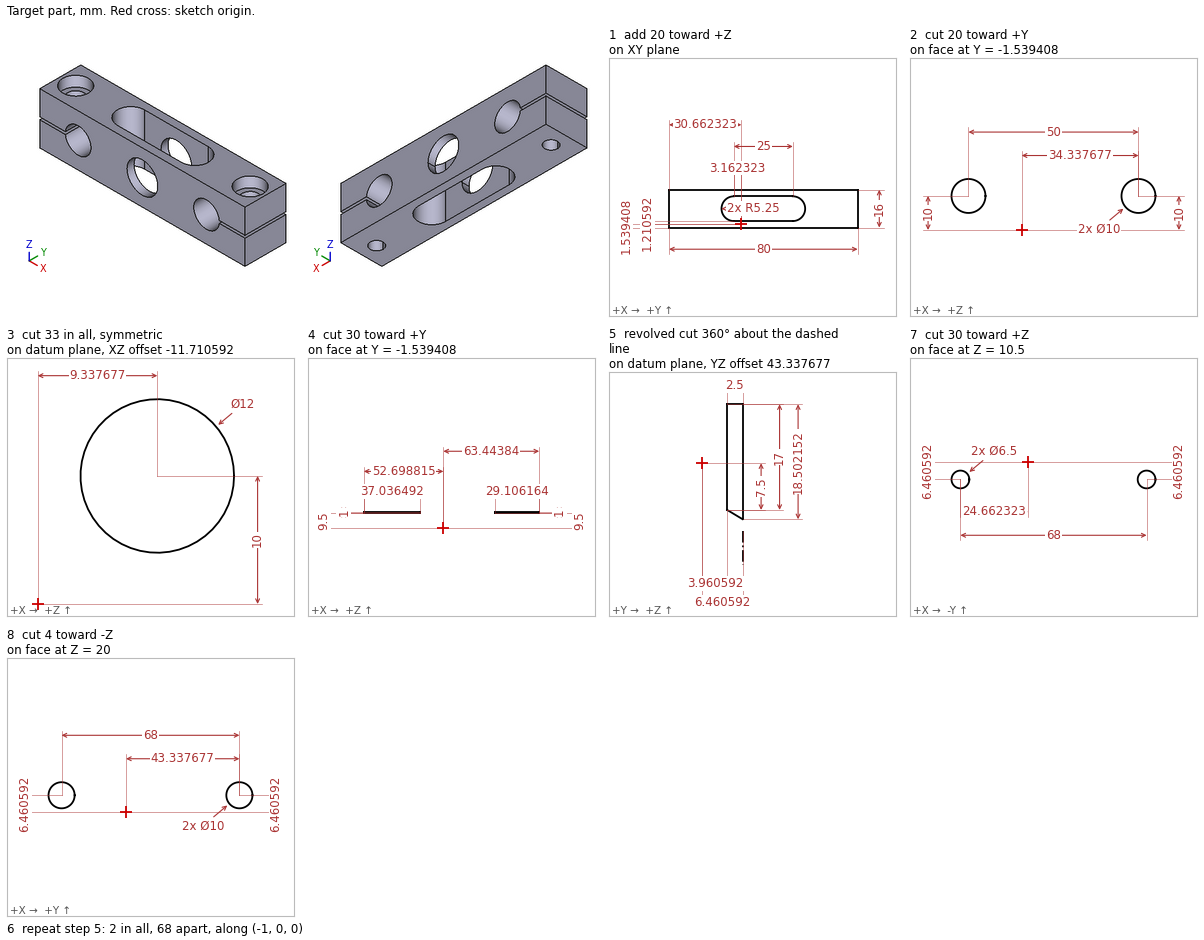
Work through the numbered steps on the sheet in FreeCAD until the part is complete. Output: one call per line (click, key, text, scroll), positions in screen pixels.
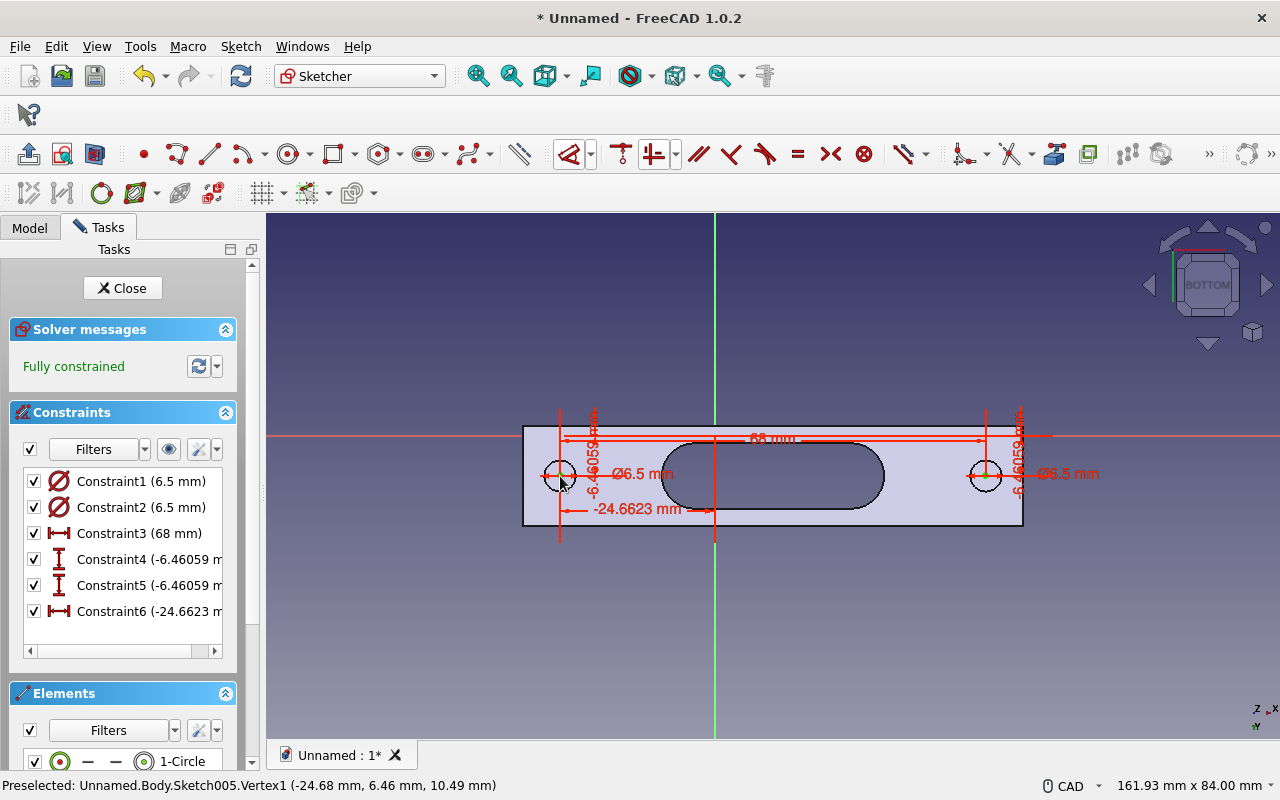
click(123, 288)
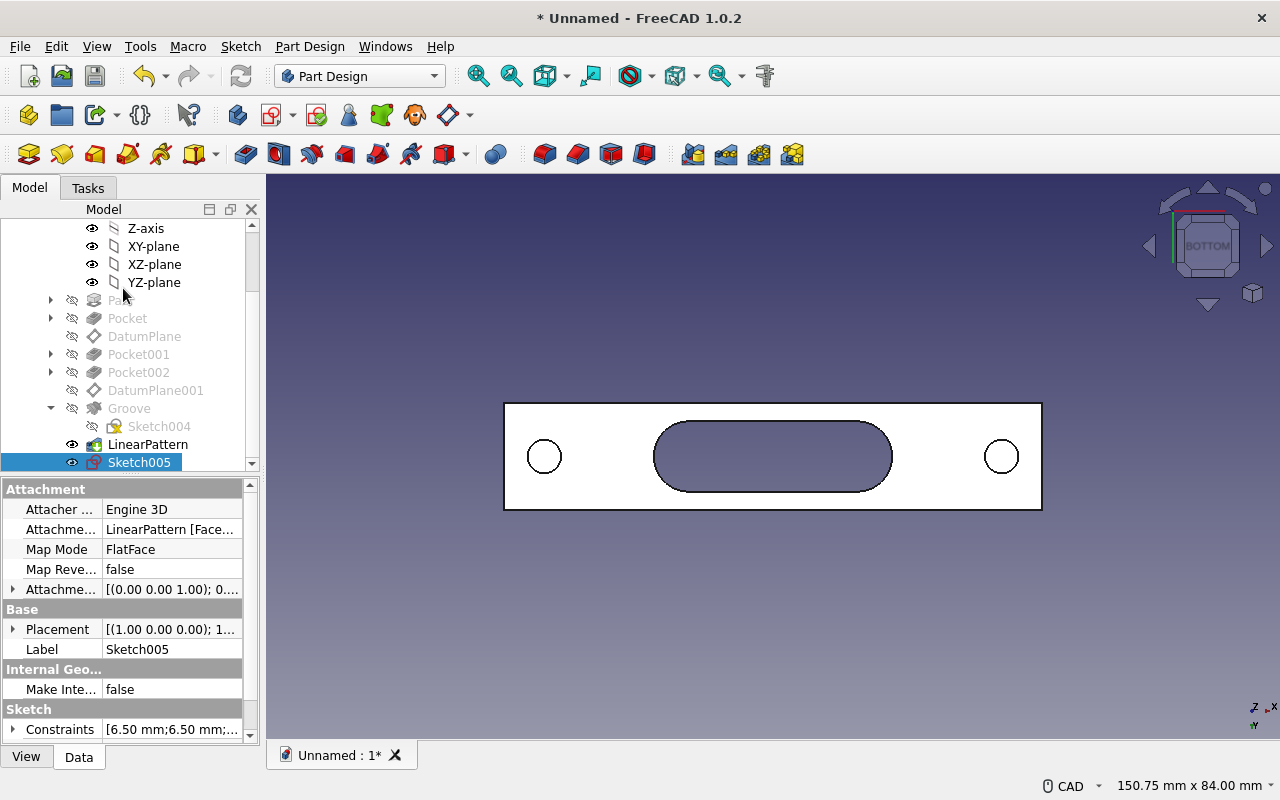
click(246, 154)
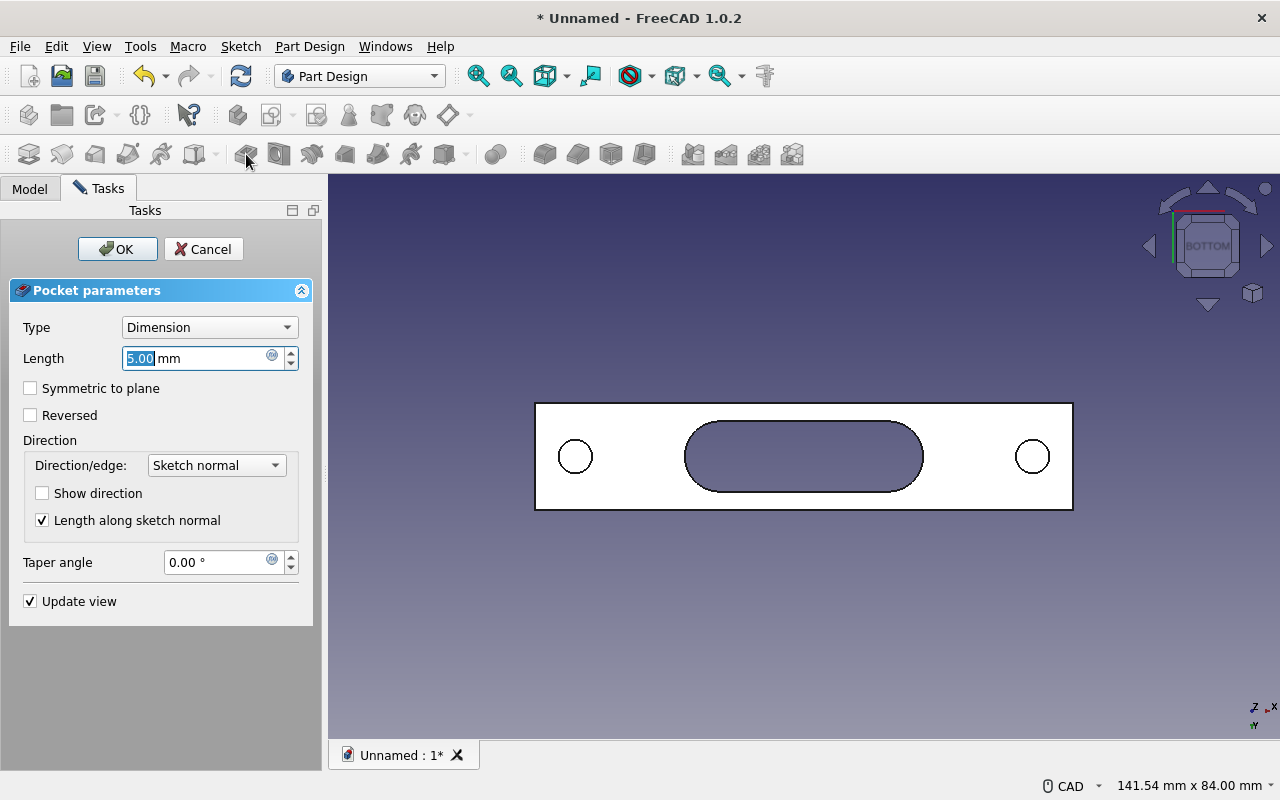
text(30)
key(Tab)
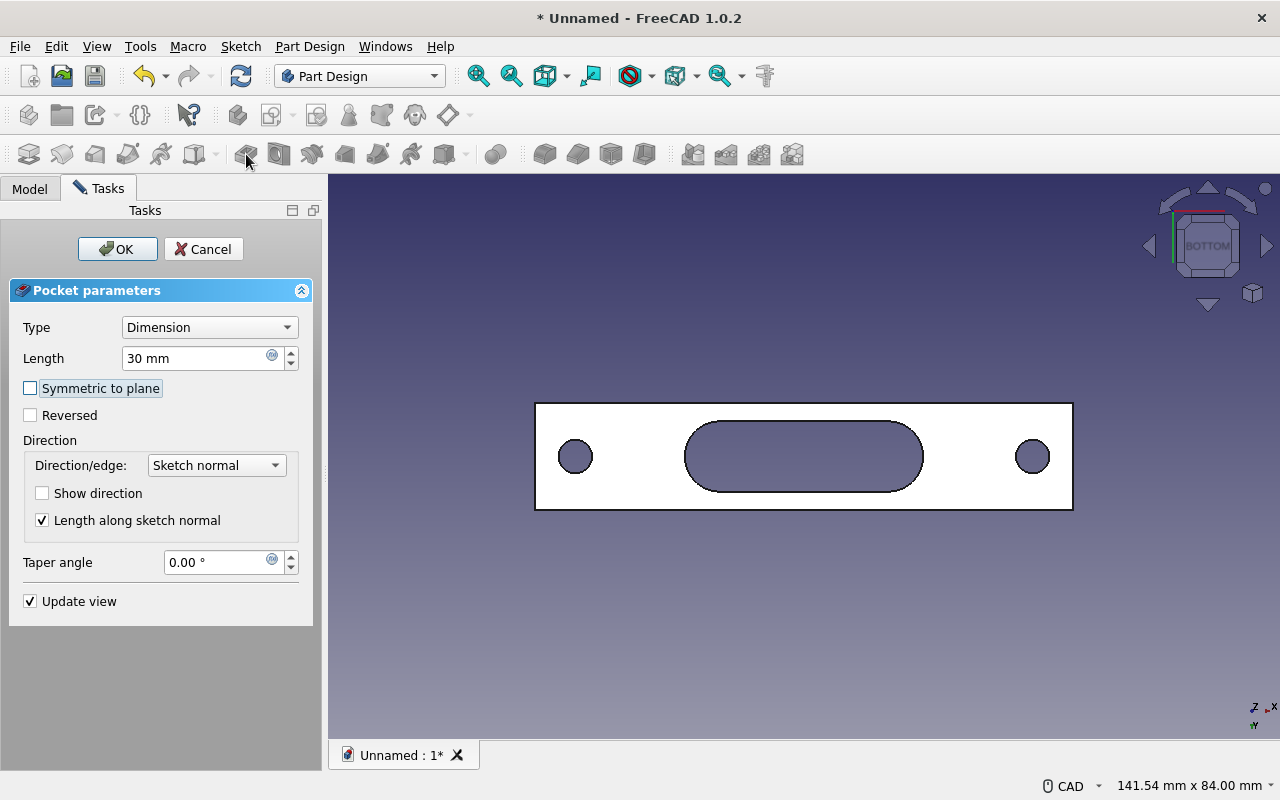
click(118, 249)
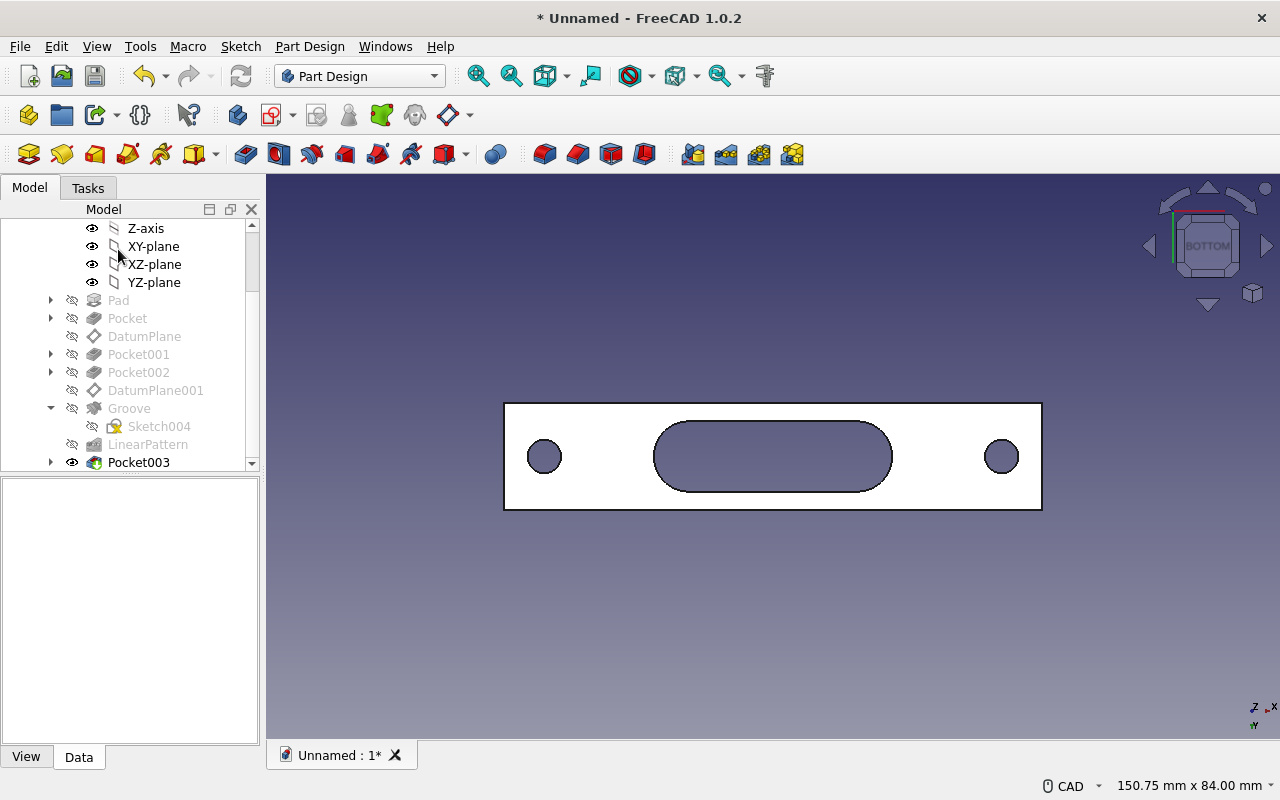
key(0)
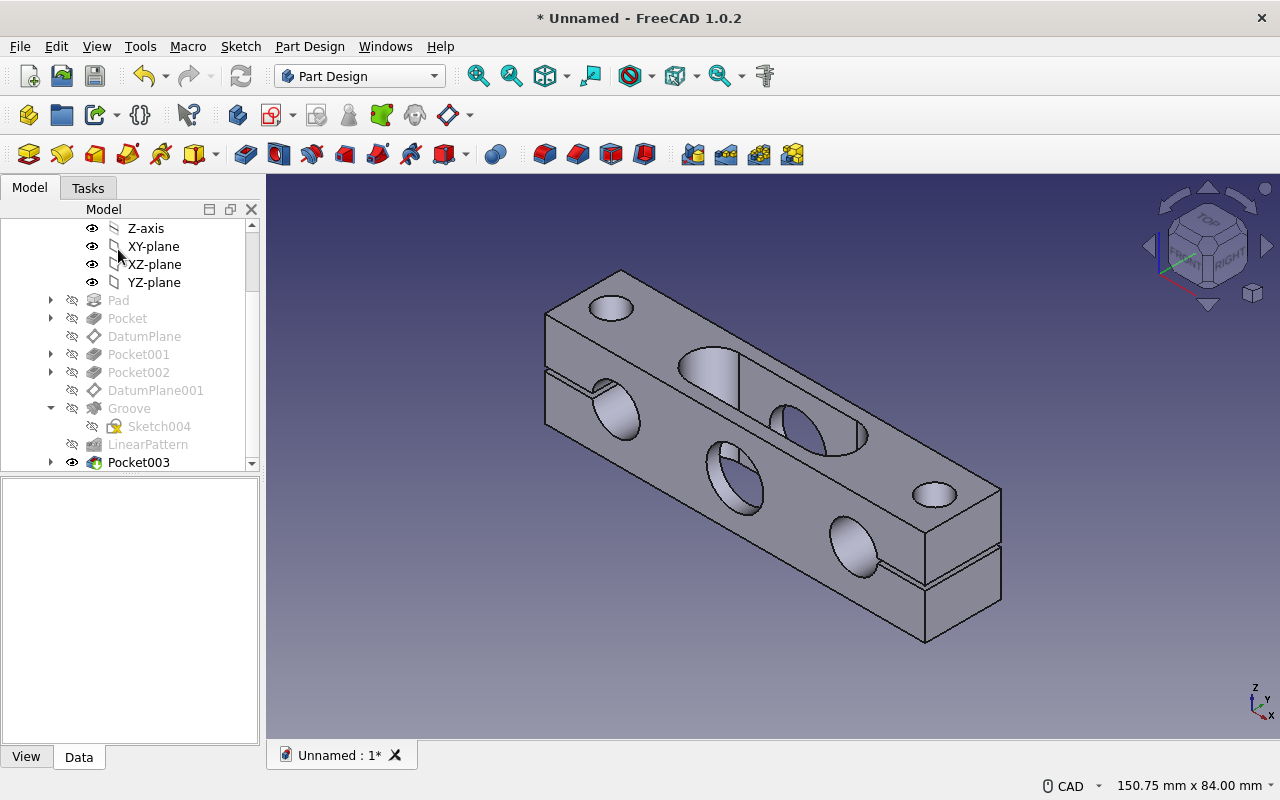
click(675, 332)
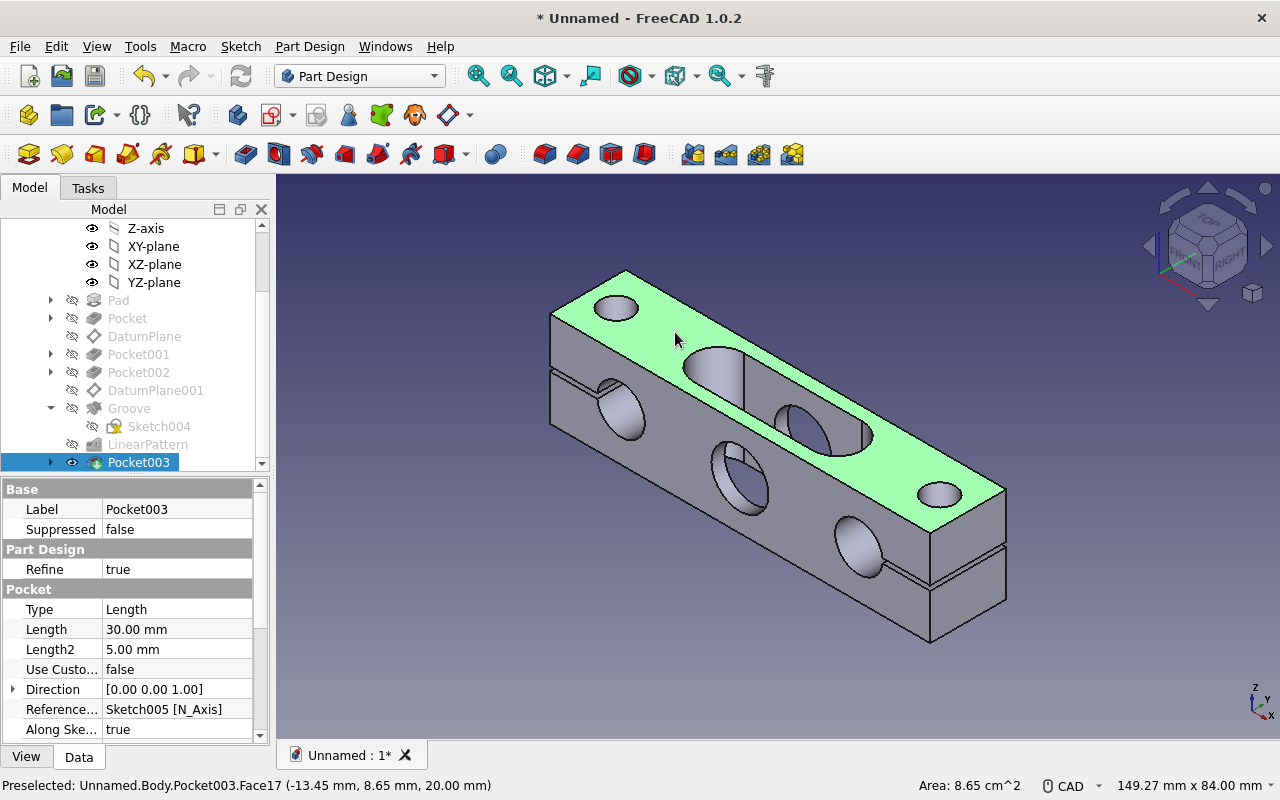
click(270, 116)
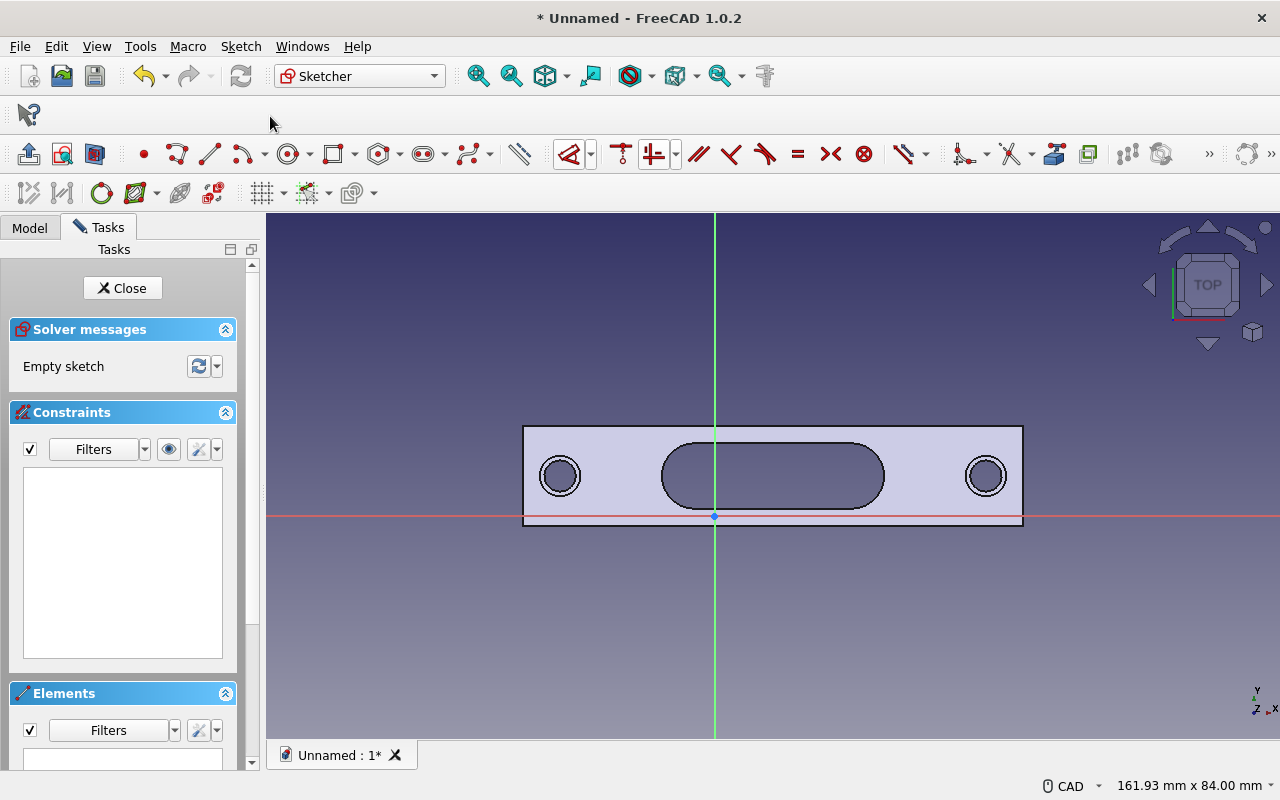
click(288, 154)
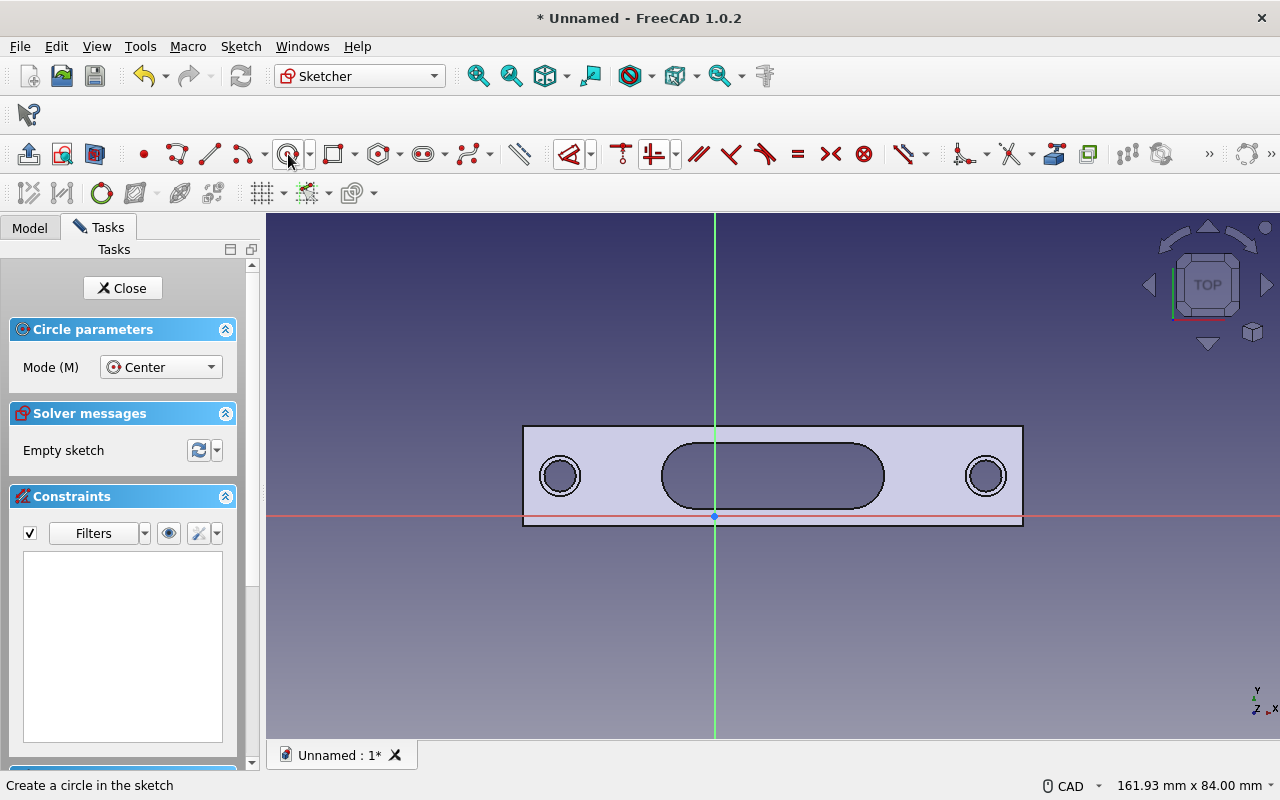
click(986, 476)
move(1008, 454)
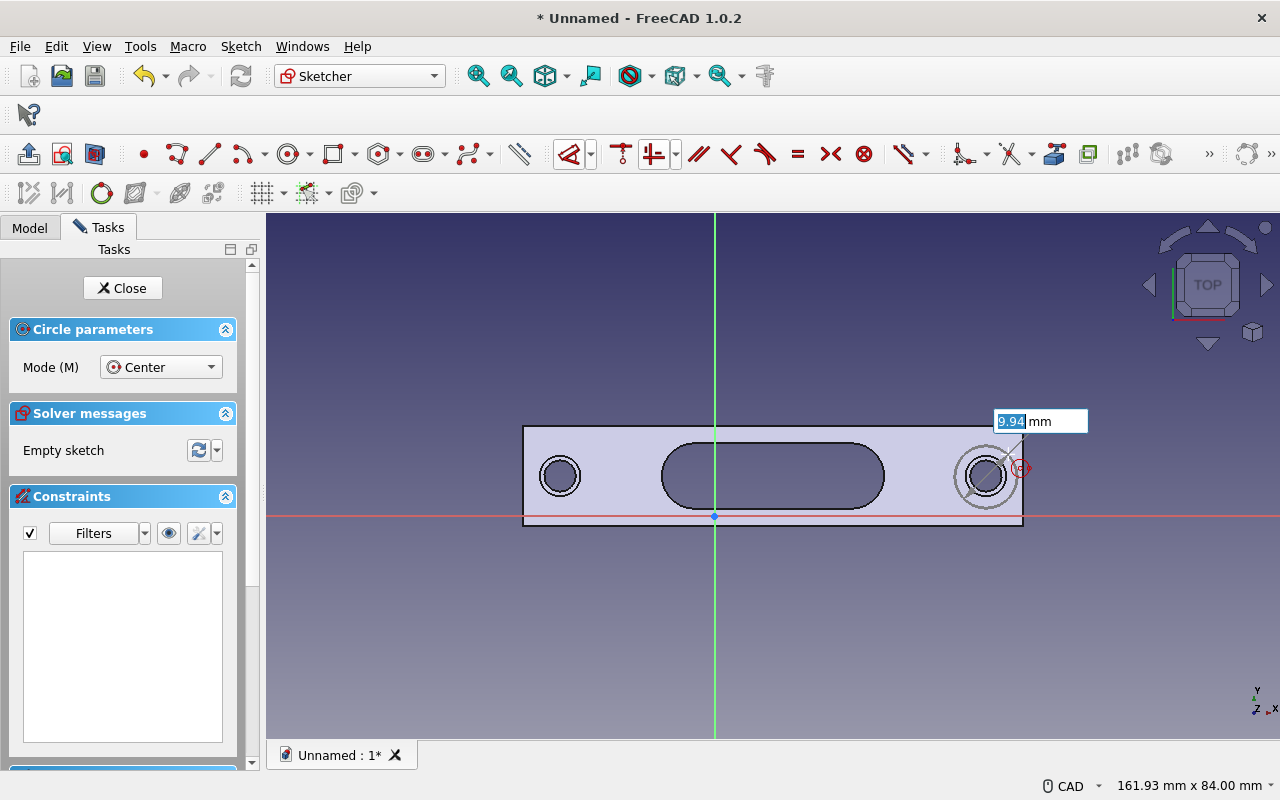
text(10)
key(Return)